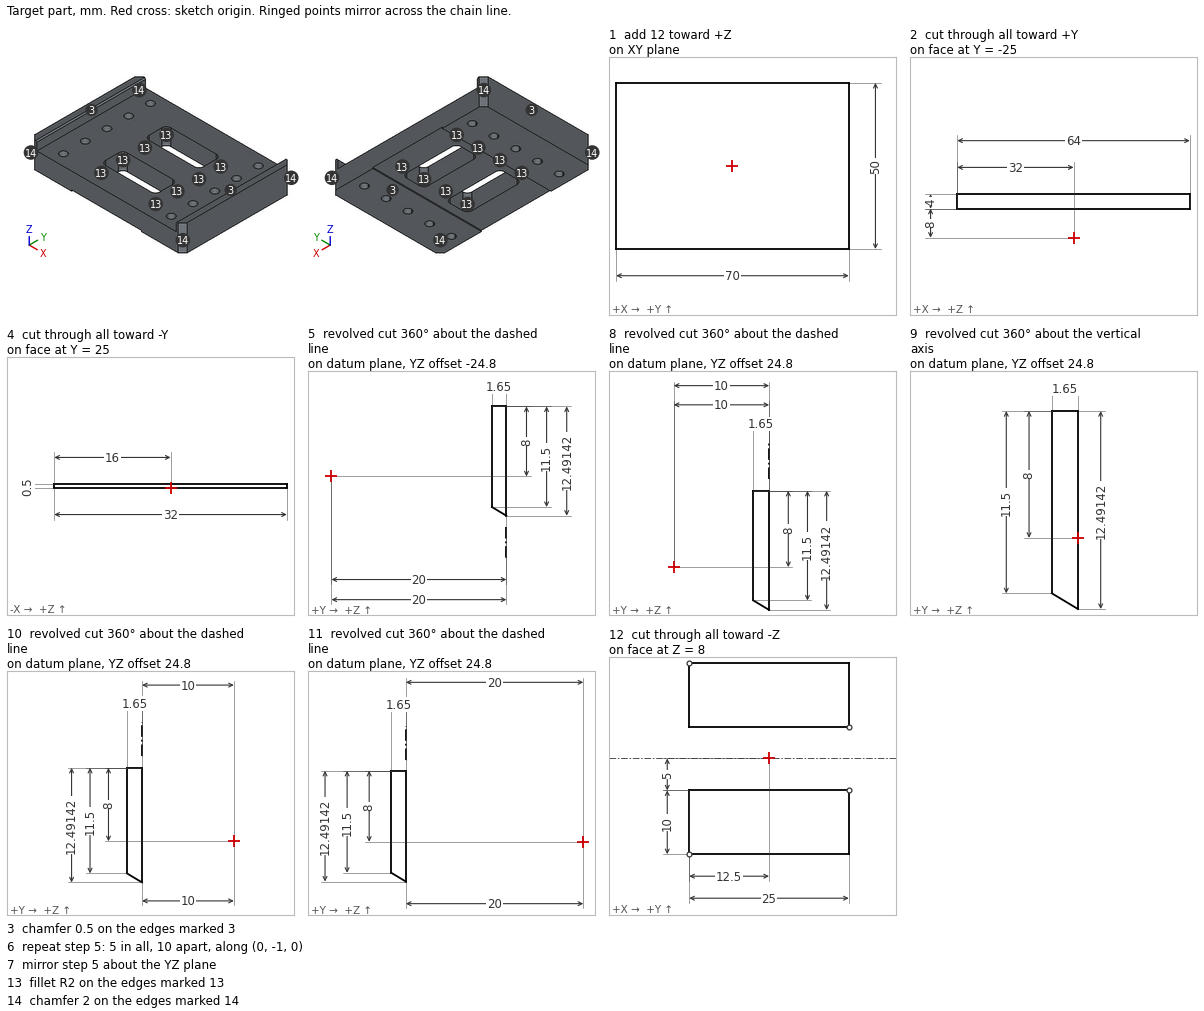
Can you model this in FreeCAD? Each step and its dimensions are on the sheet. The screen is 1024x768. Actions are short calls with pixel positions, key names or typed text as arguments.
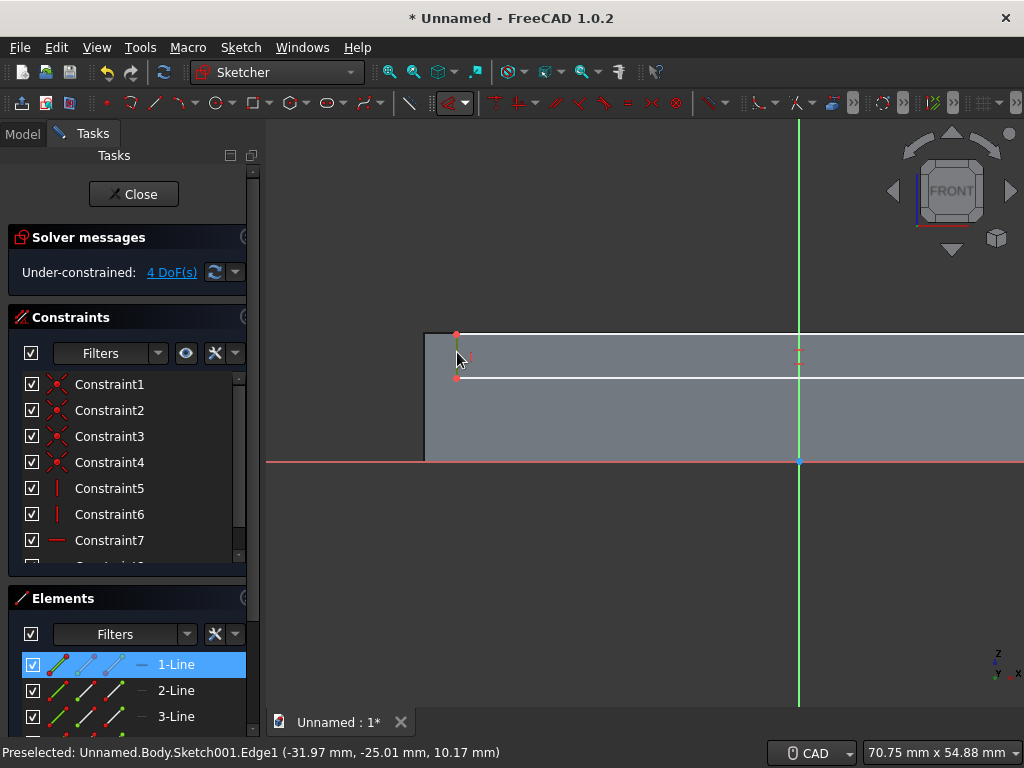
key(i)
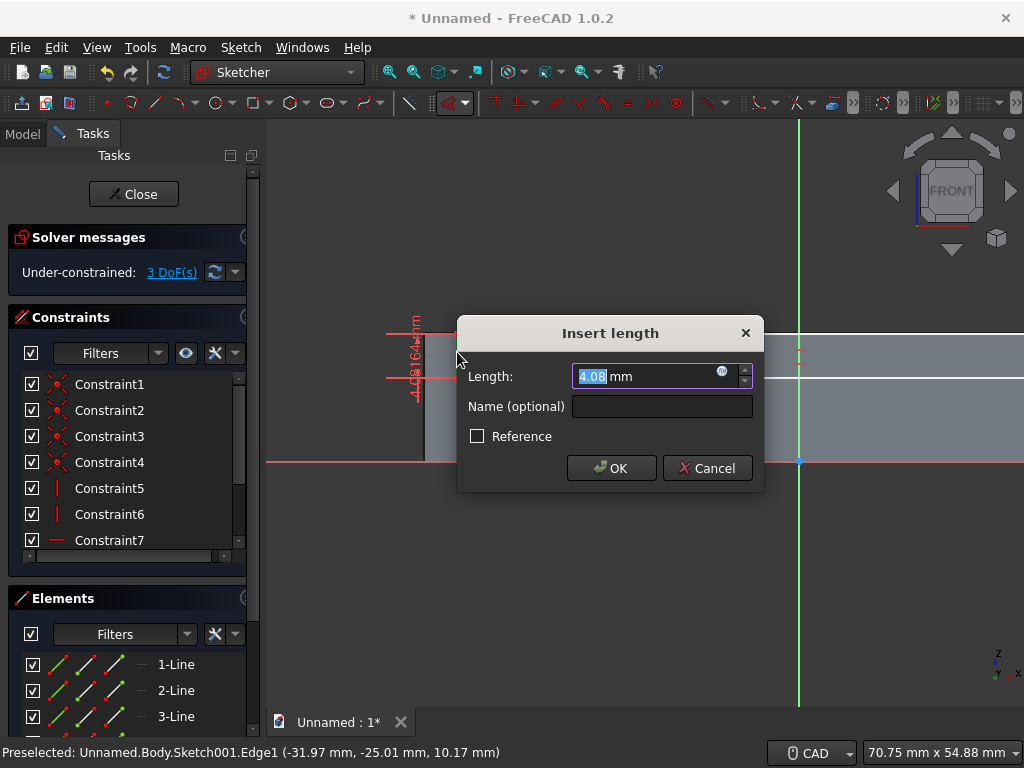
text(4)
key(Return)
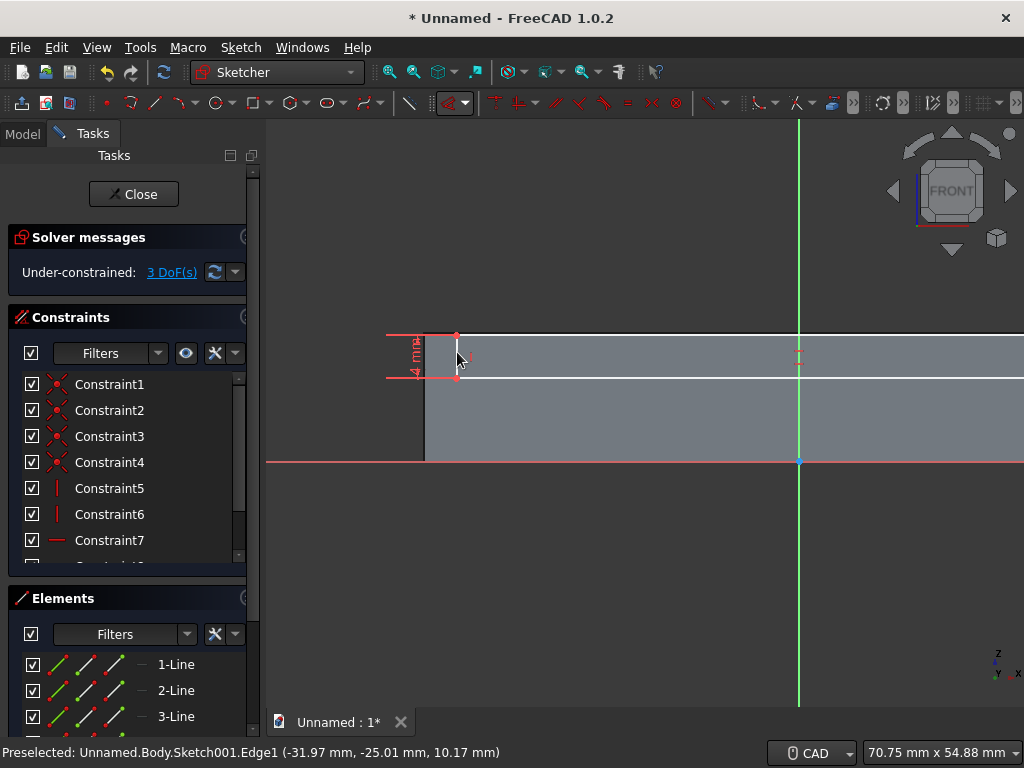
click(662, 378)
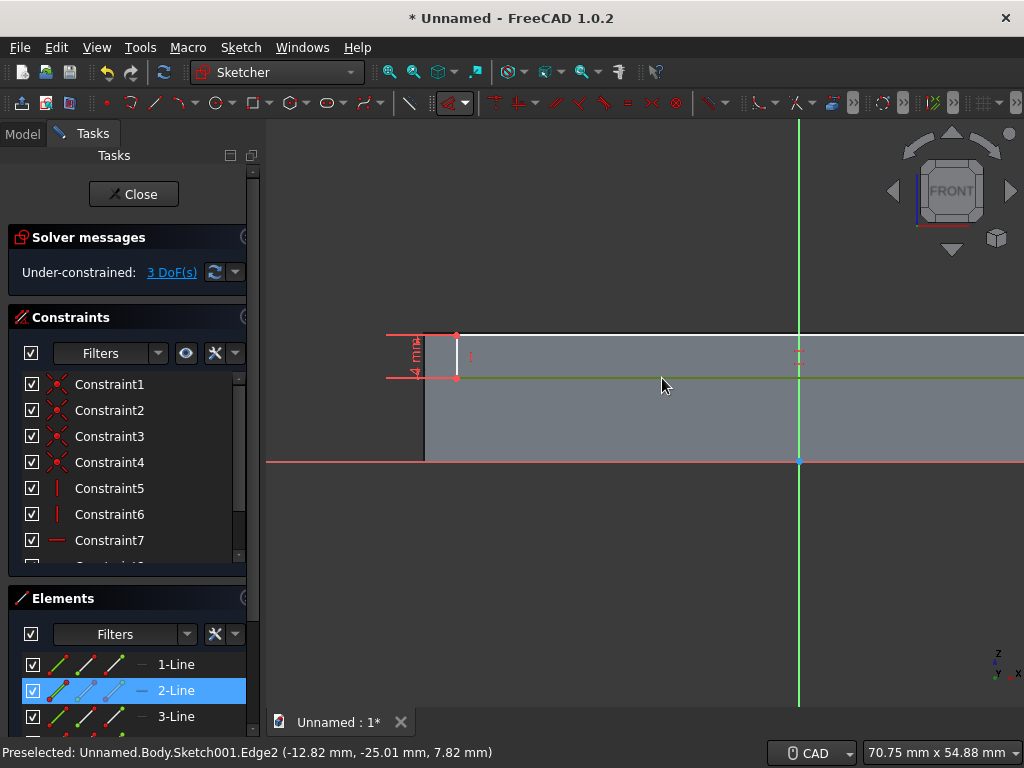
key(l)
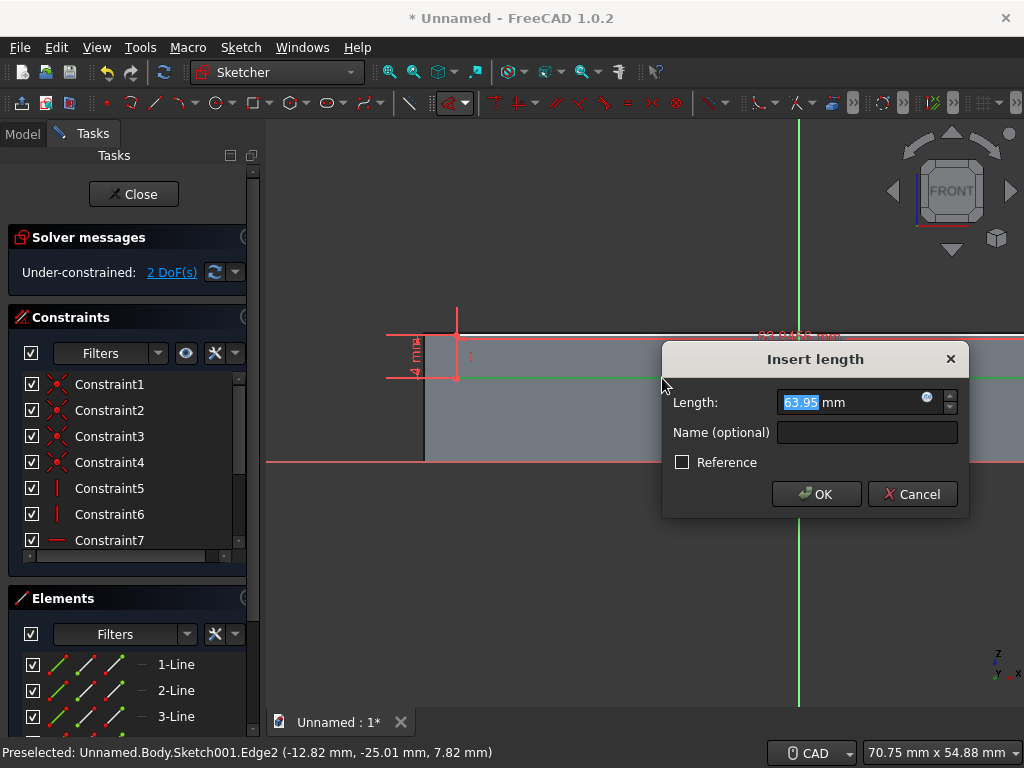
text(64)
key(Return)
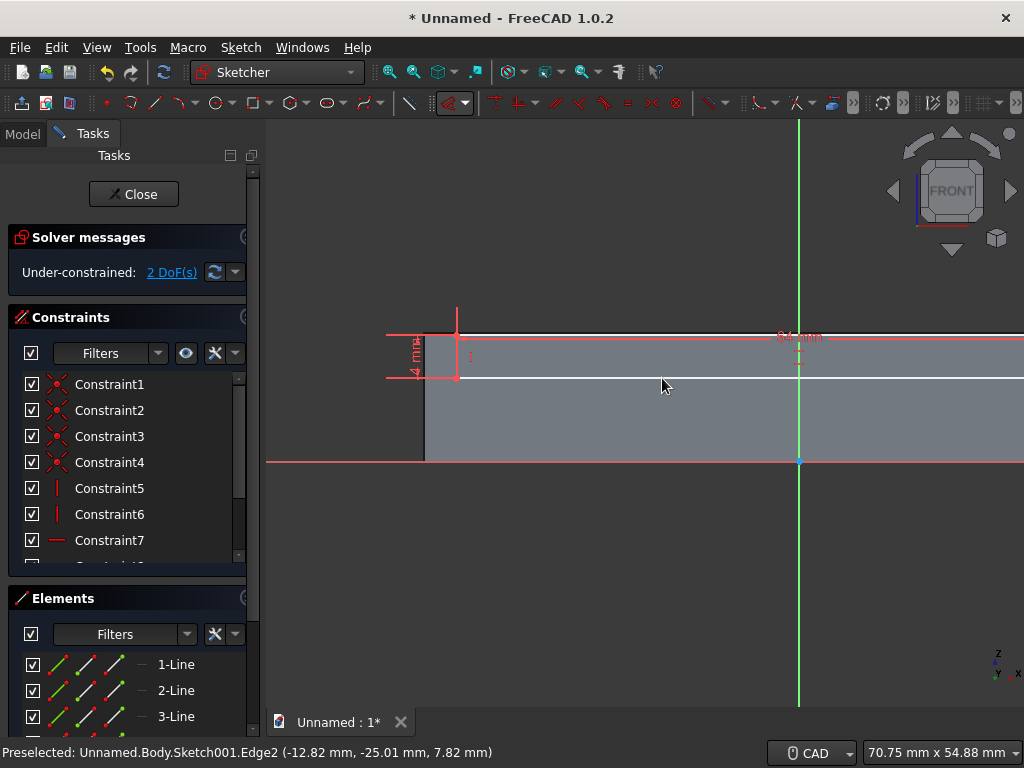
click(457, 378)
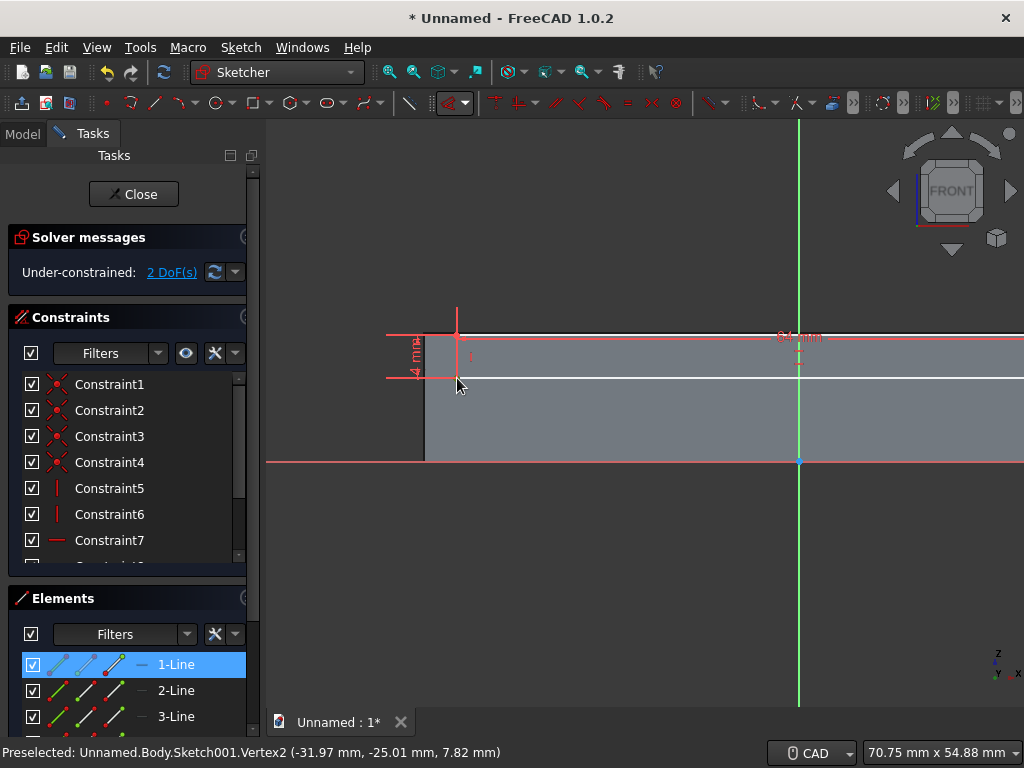
key(i)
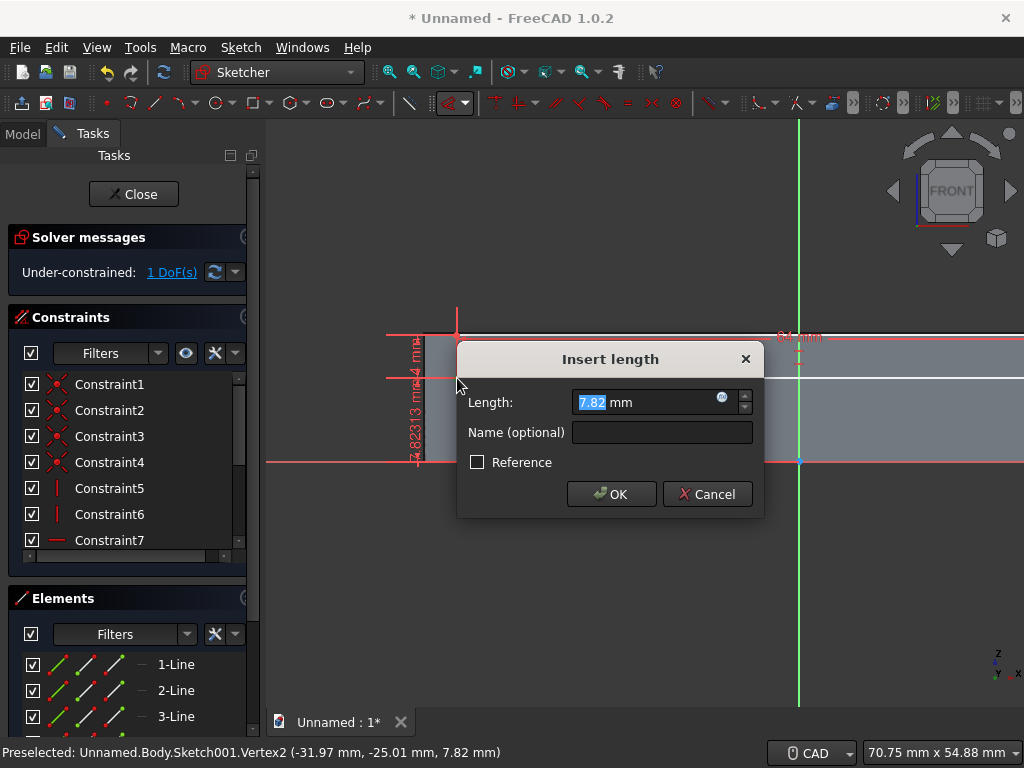
text(8)
key(Return)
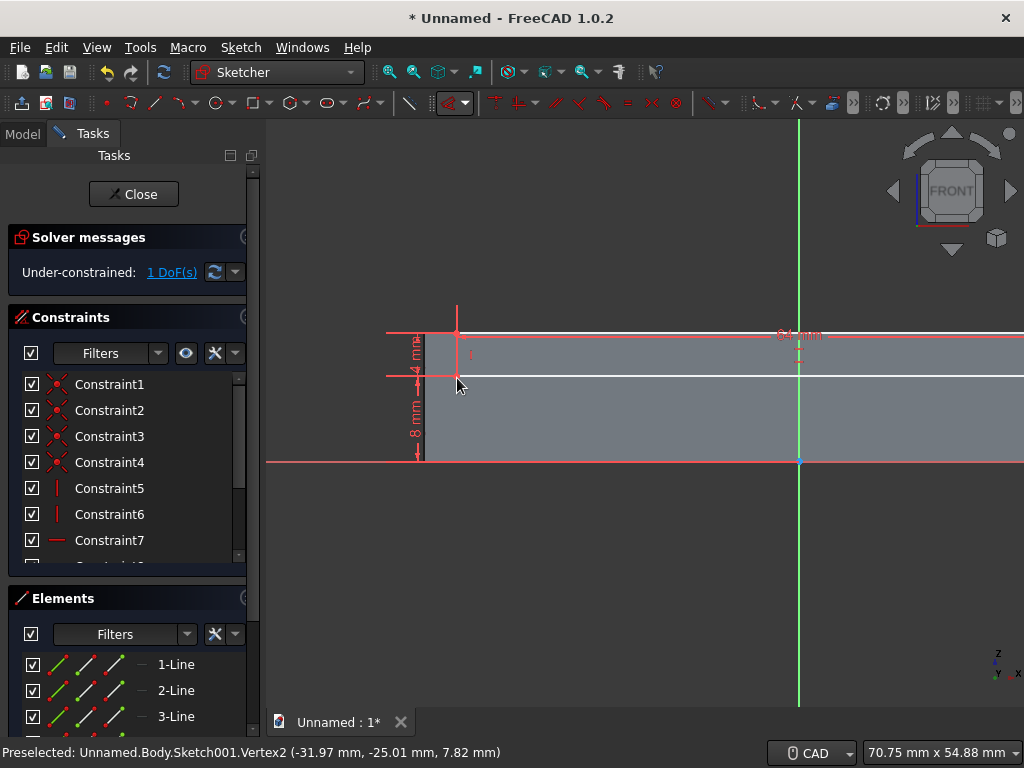
click(457, 333)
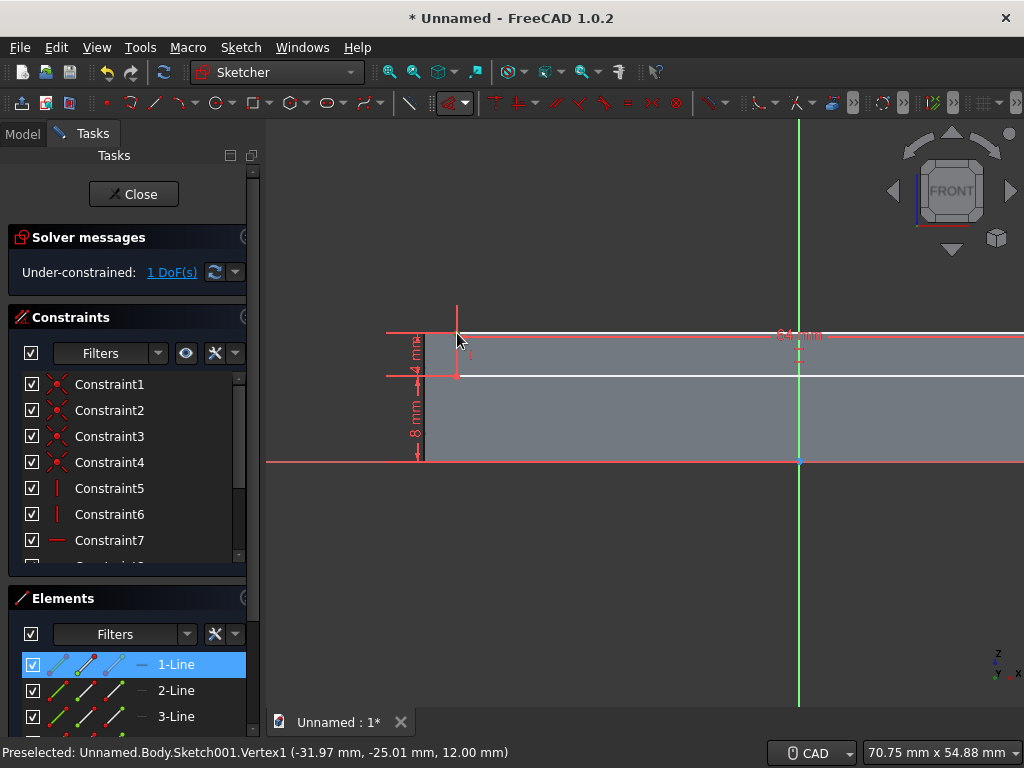
key(l)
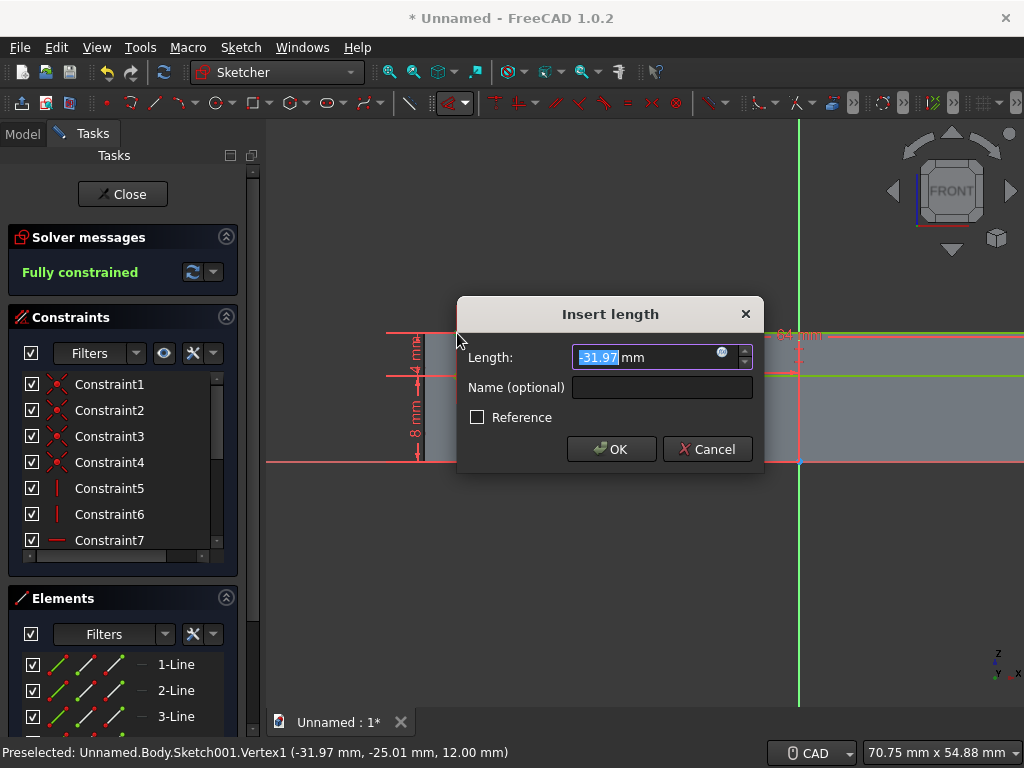
text(-32)
key(Return)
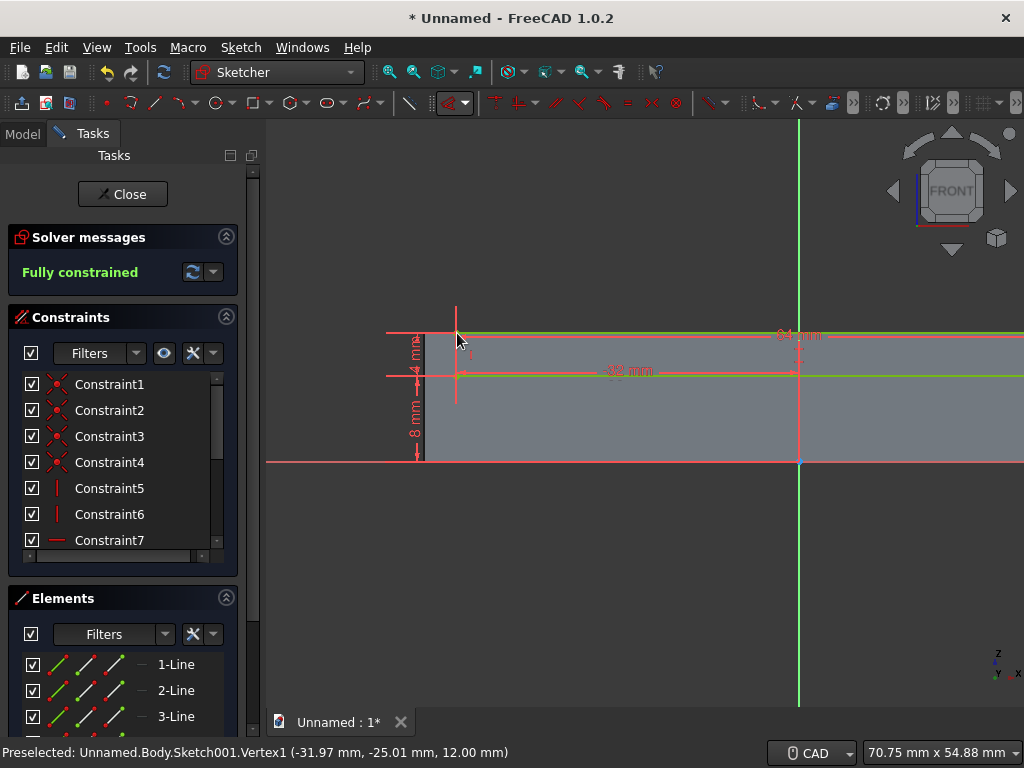
click(123, 194)